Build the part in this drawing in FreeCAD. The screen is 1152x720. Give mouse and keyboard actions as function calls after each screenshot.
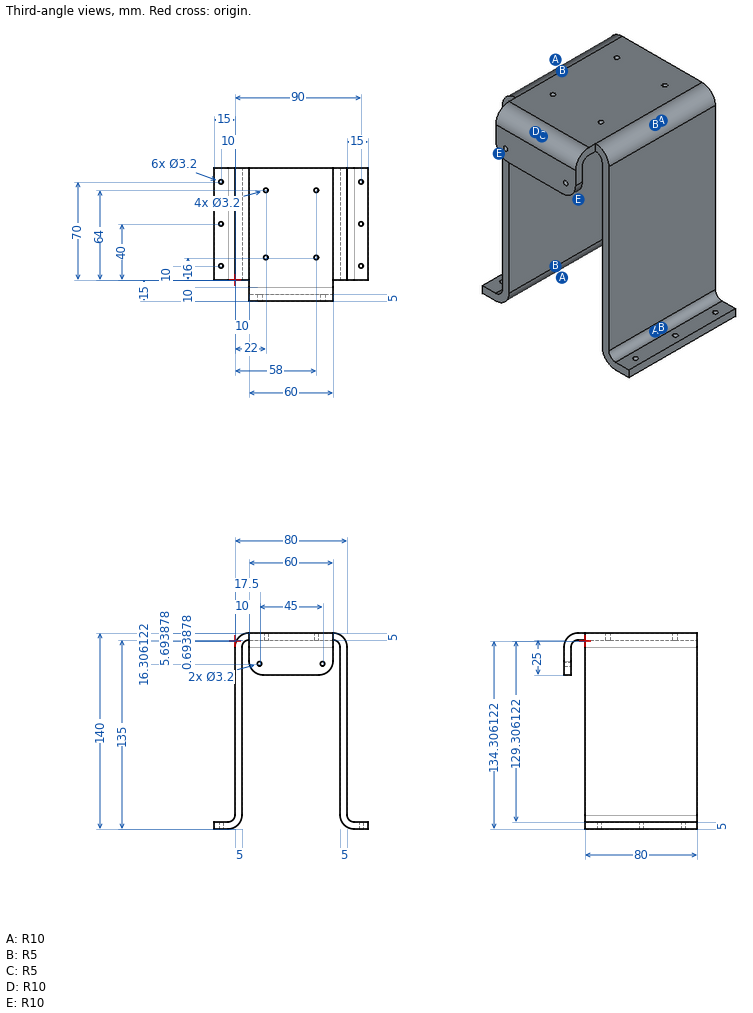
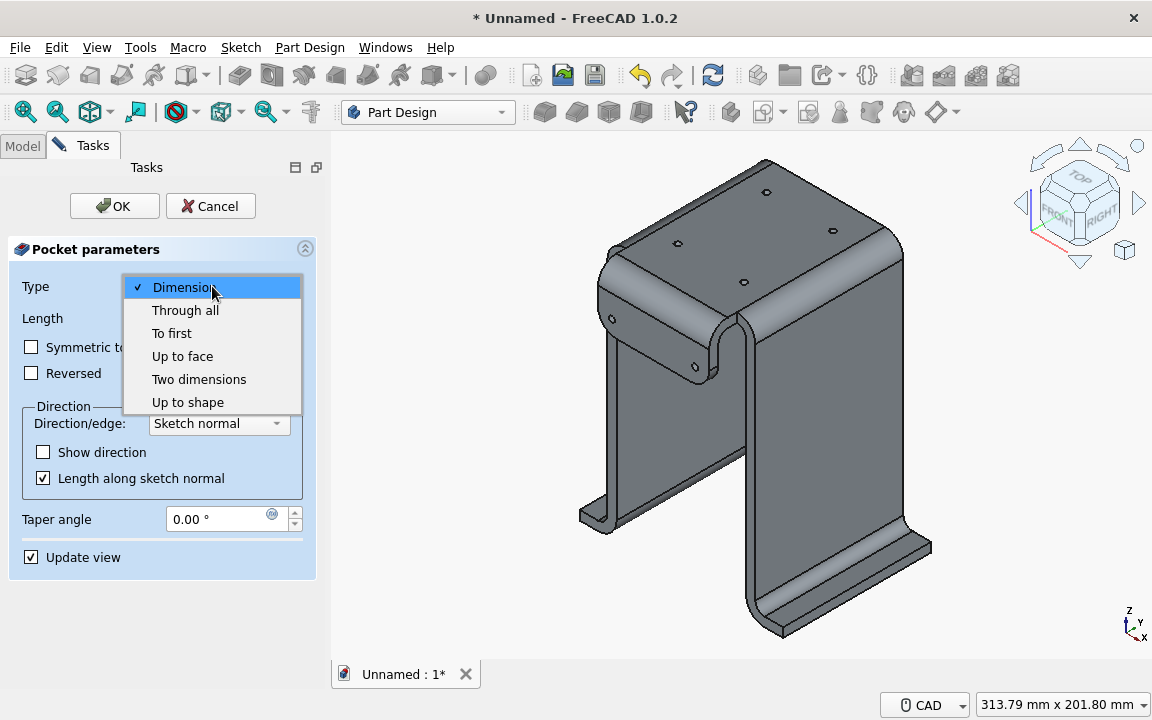
click(212, 310)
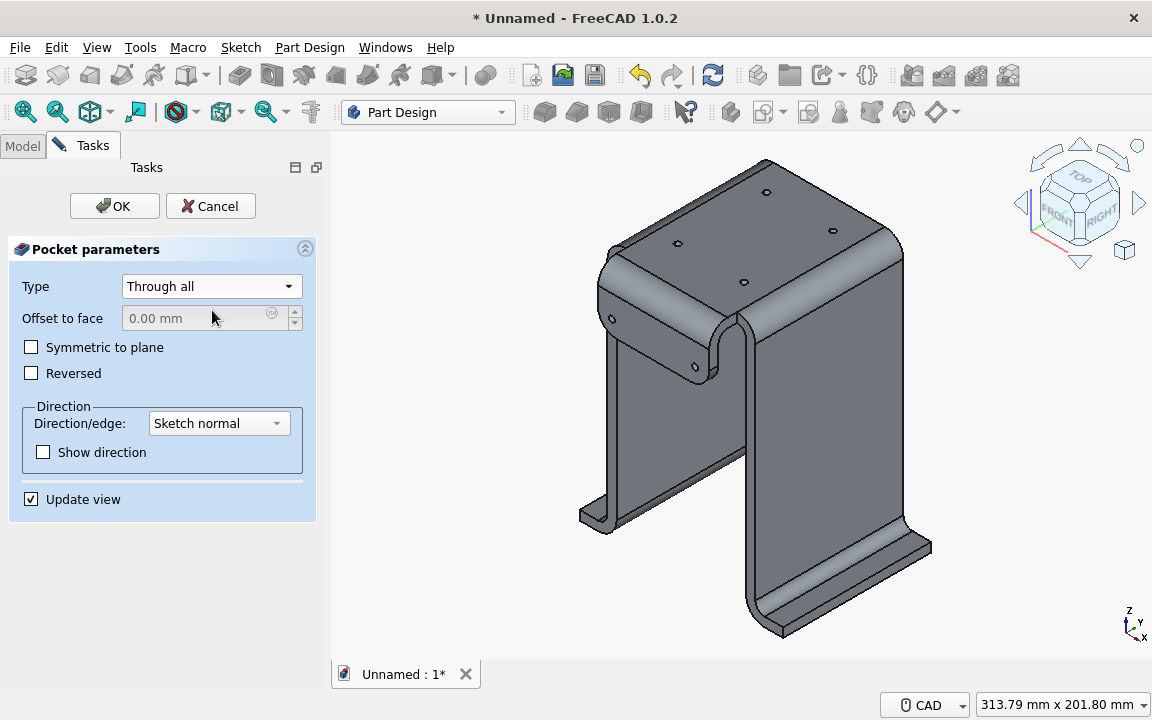
click(115, 206)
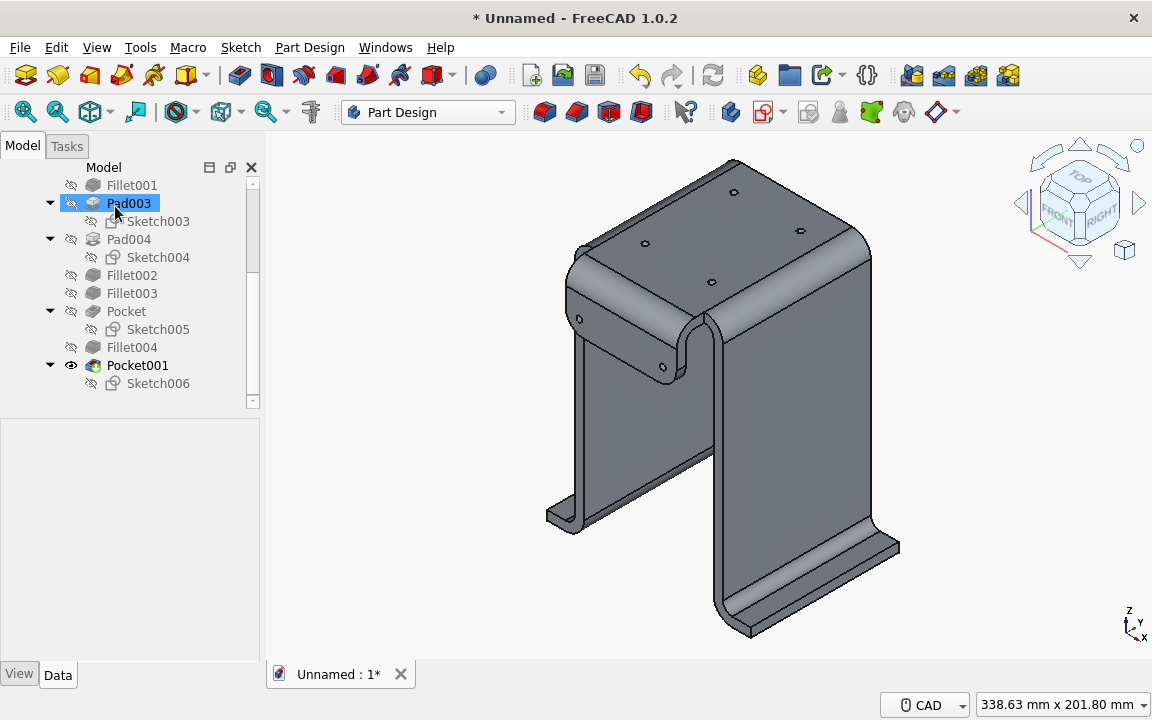
key(2)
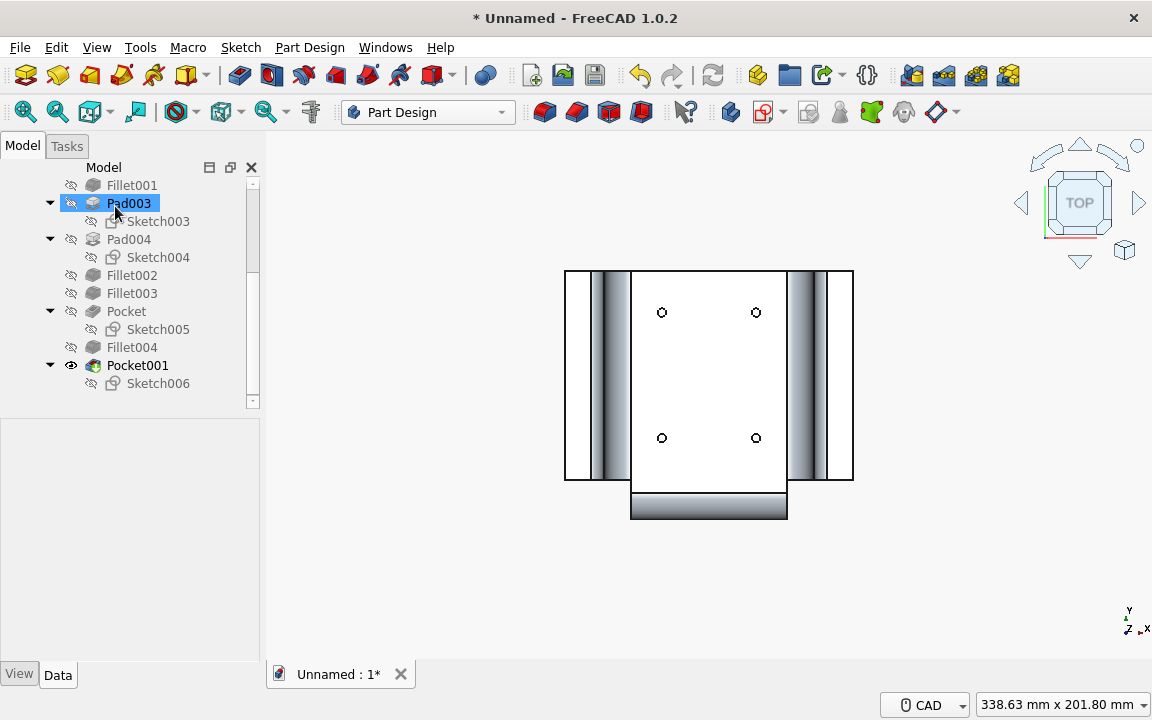
click(578, 285)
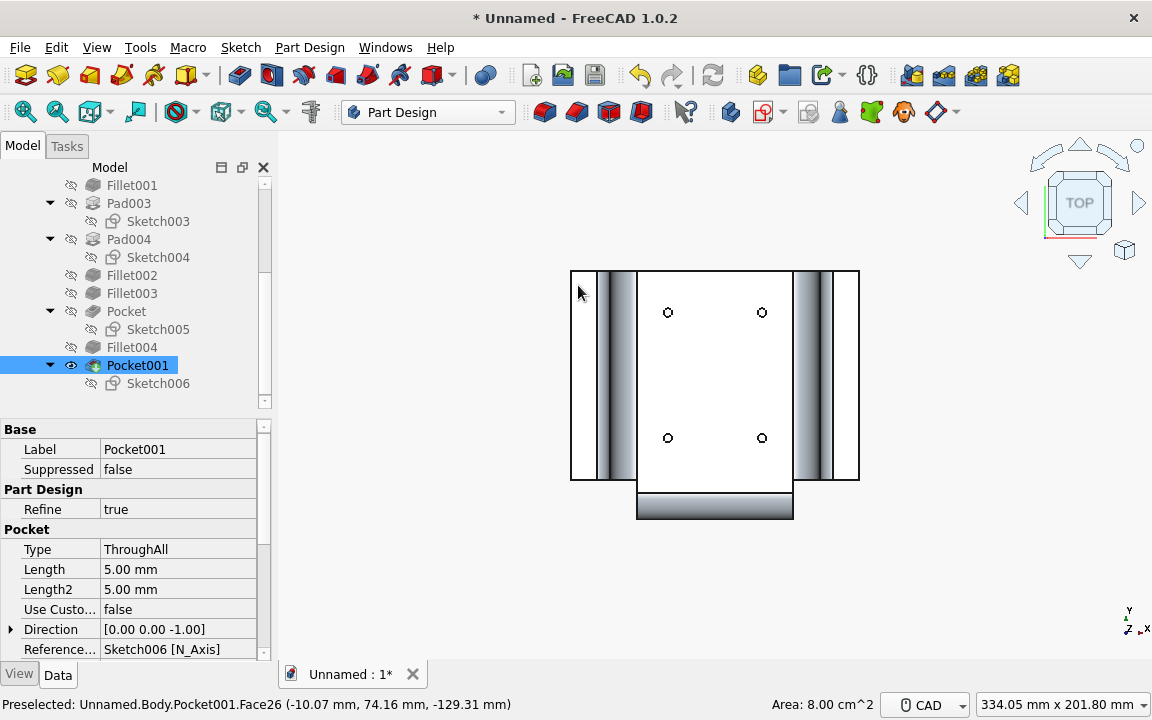
click(764, 112)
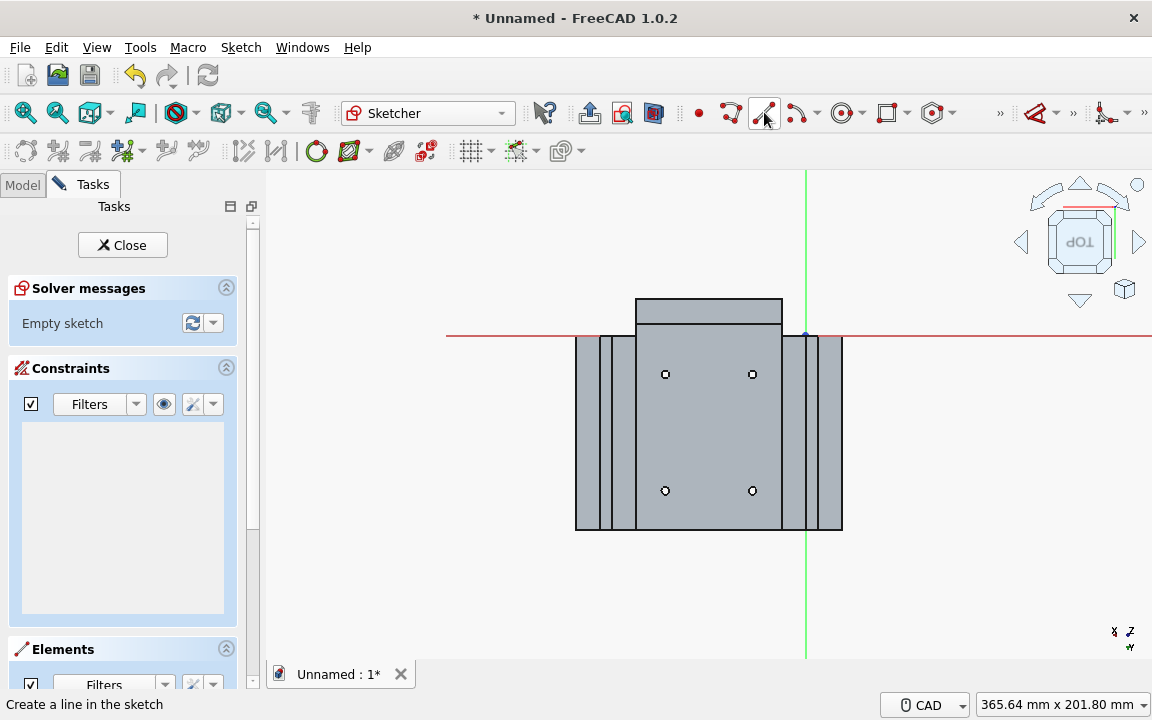
click(654, 114)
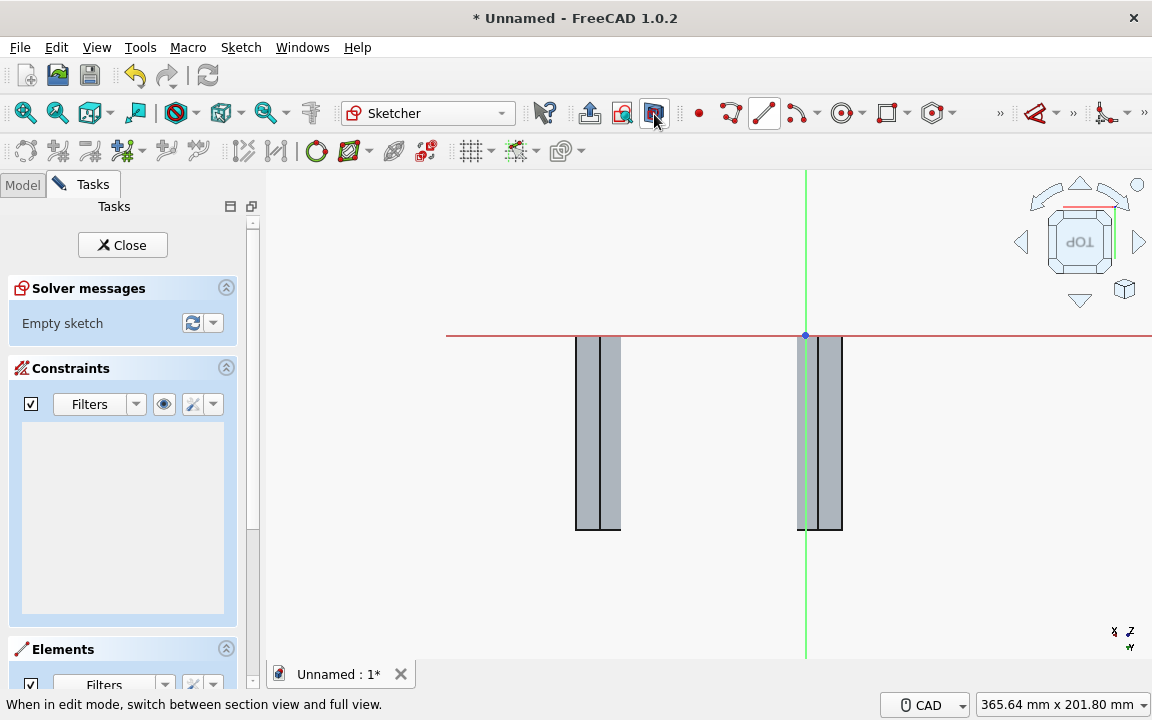
scroll(792, 432, up, 3)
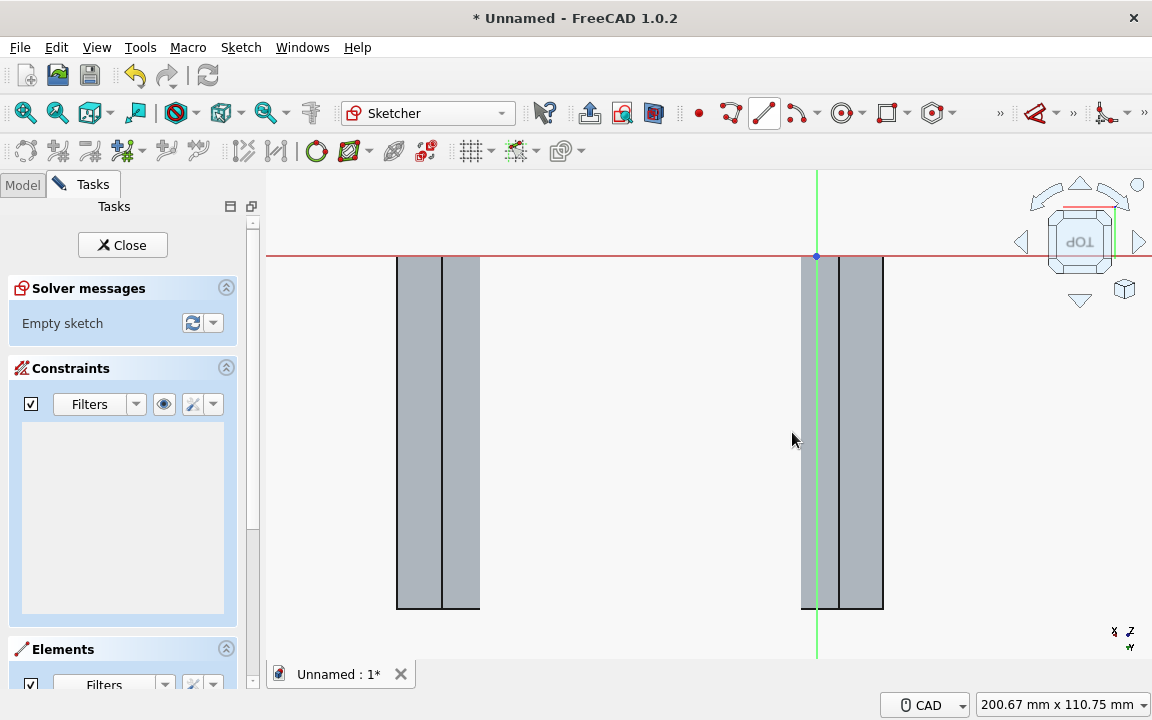
click(842, 114)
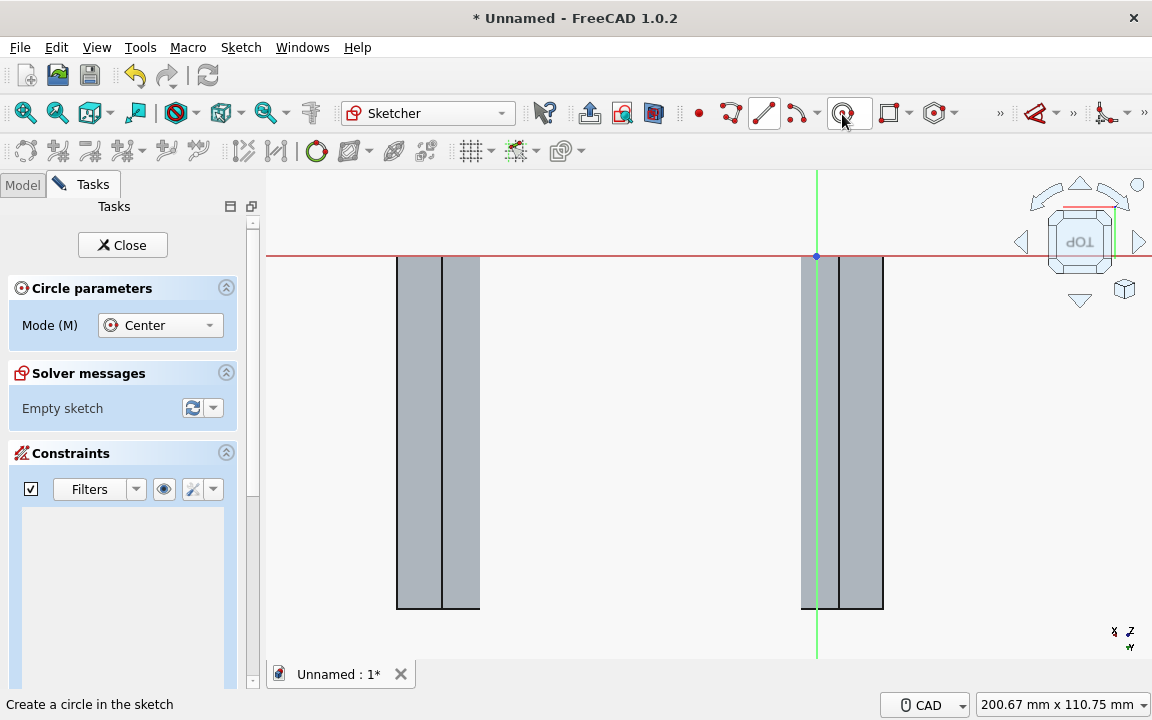
scroll(861, 565, up, 6)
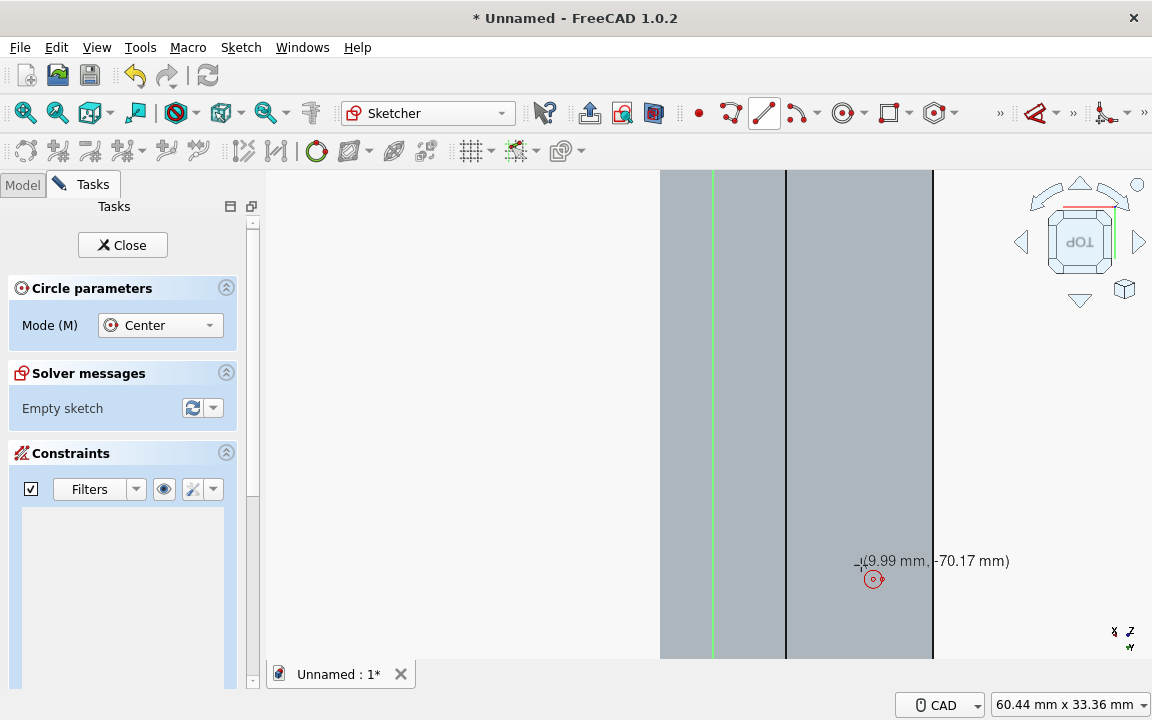
click(860, 564)
move(876, 547)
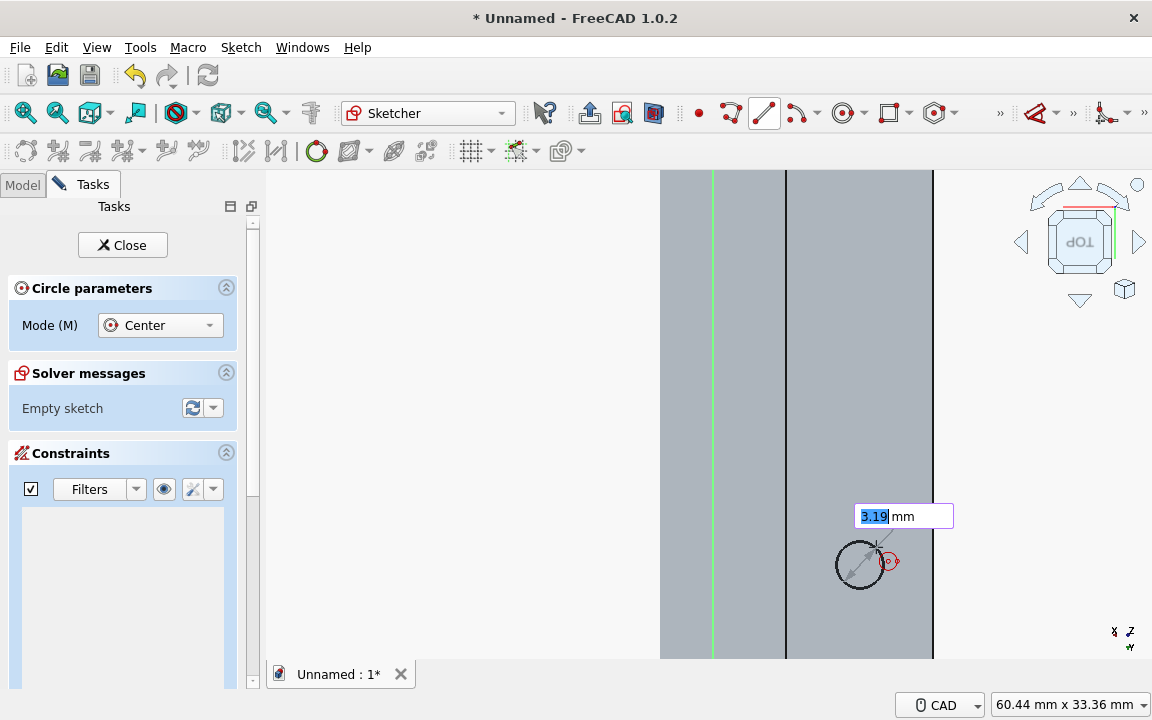
text(3.2)
key(Return)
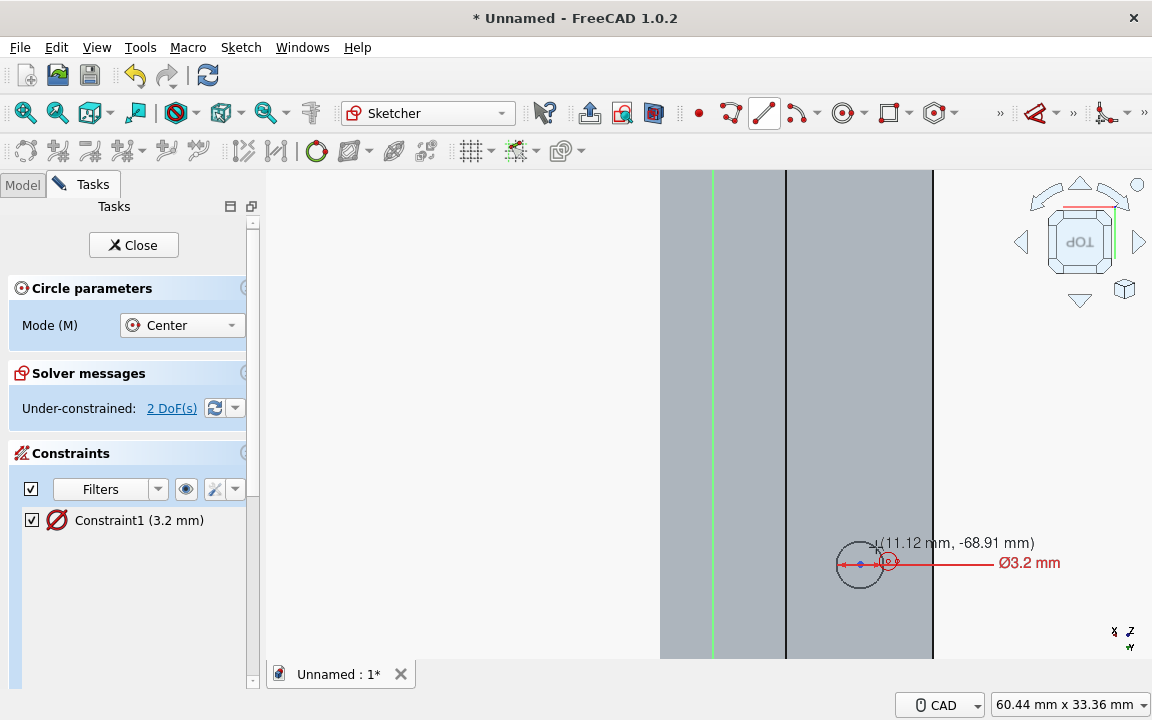
scroll(862, 566, down, 6)